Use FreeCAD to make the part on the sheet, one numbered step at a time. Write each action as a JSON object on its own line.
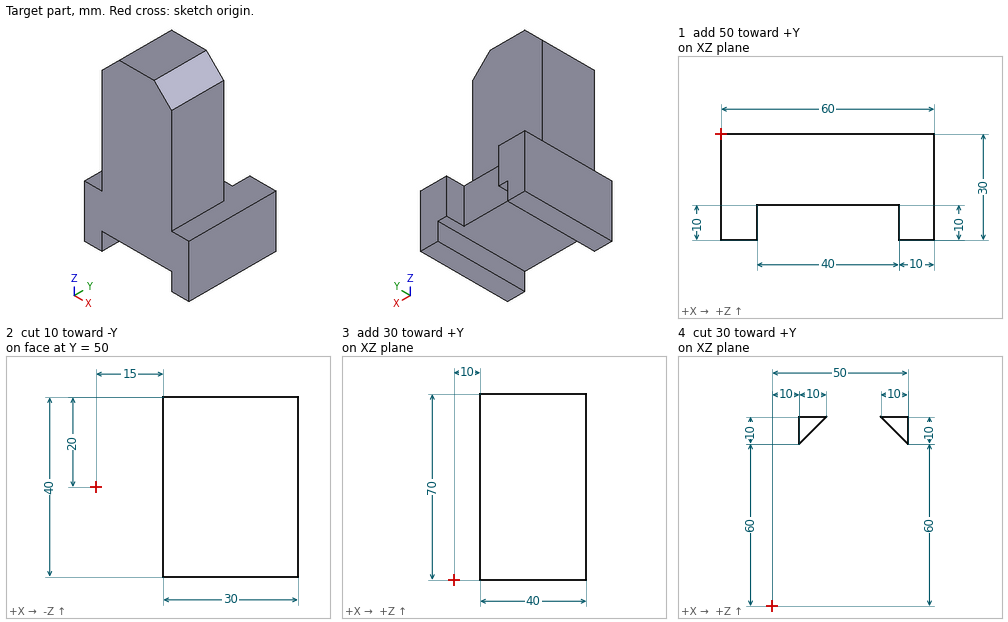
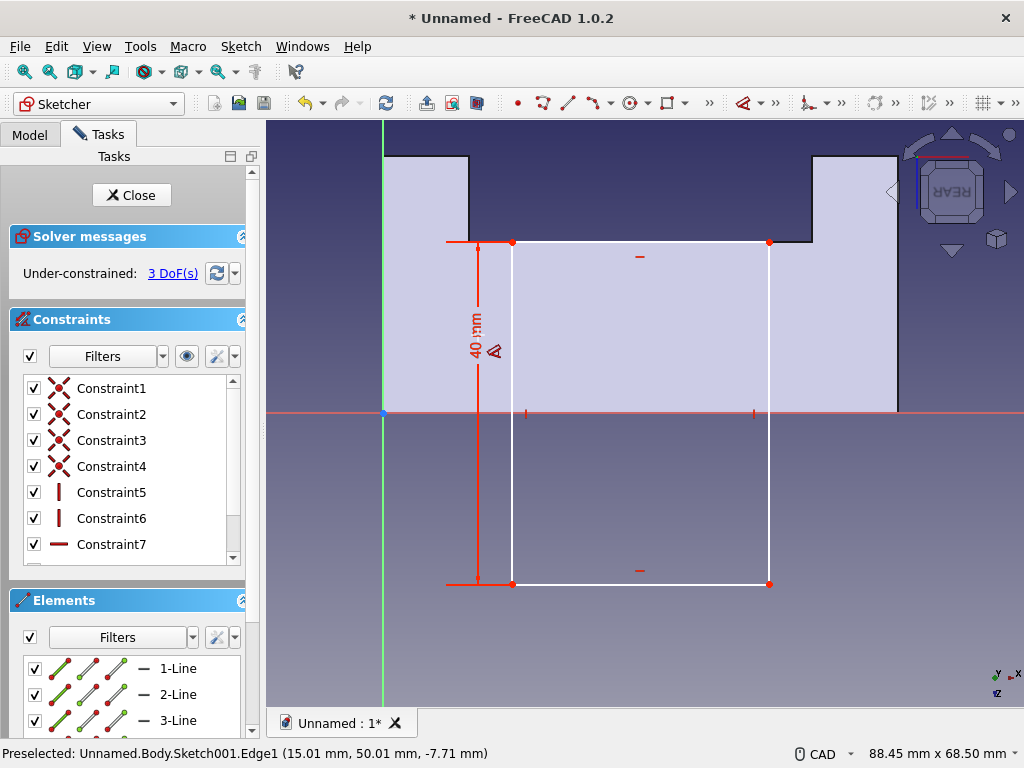
{"action": "left_click", "coordinate": [589, 585]}
{"action": "left_click", "coordinate": [641, 619]}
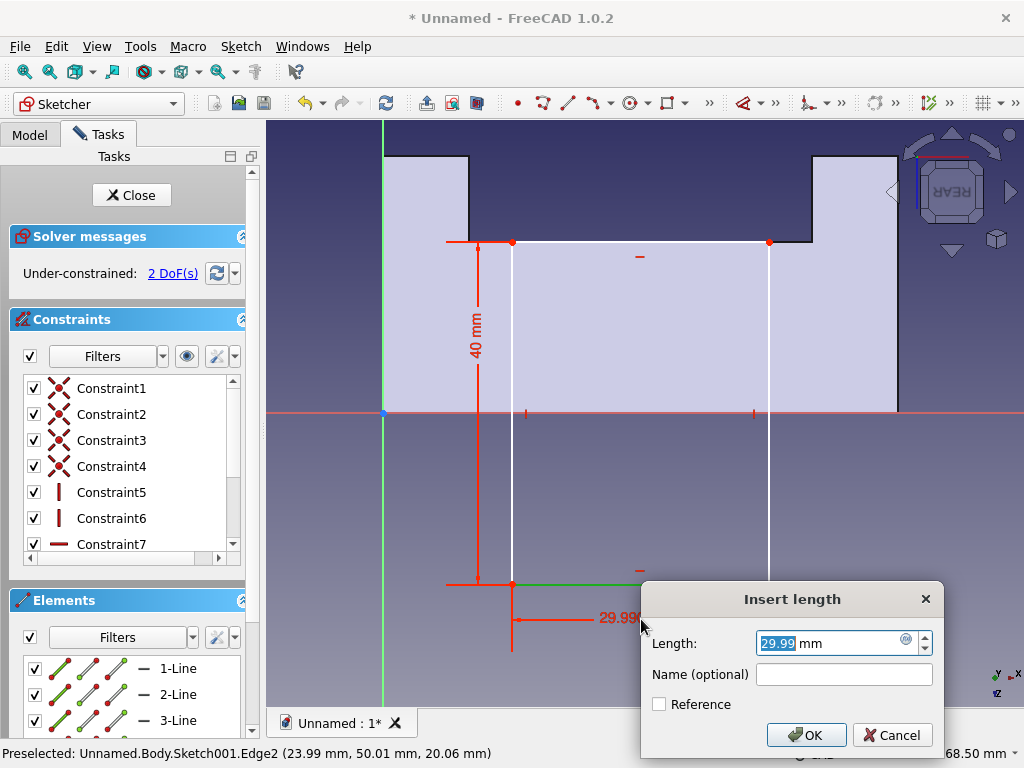
{"action": "type", "text": "30"}
{"action": "key", "text": "Return"}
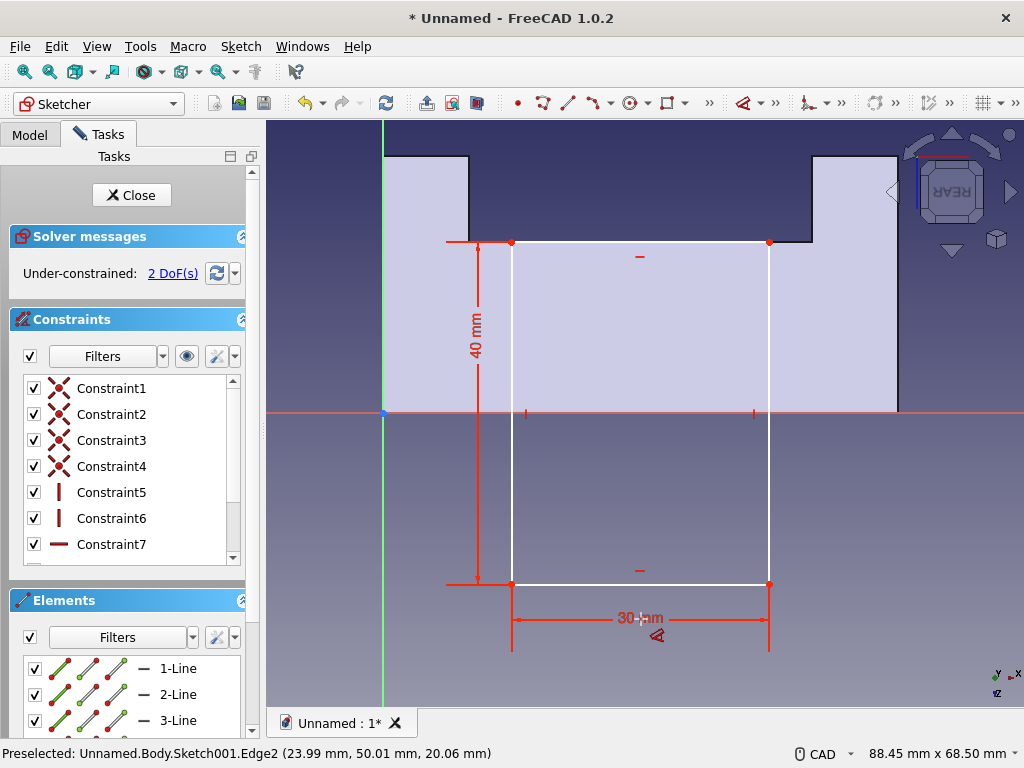
{"action": "left_click", "coordinate": [512, 242]}
{"action": "left_click", "coordinate": [448, 208]}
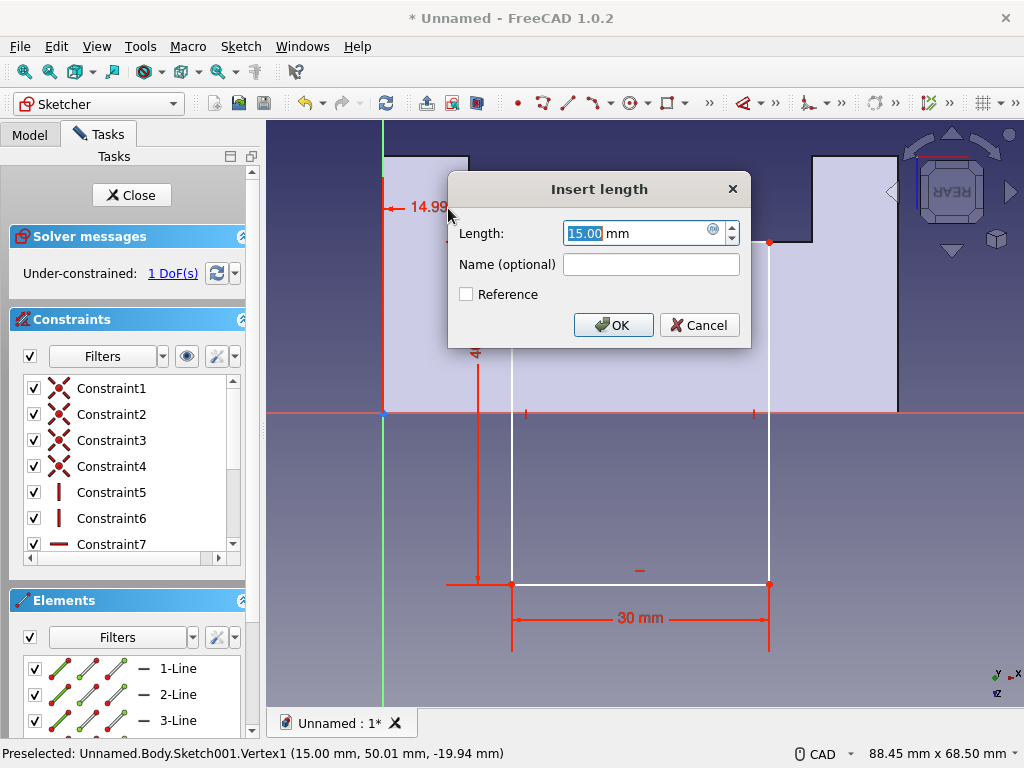
{"action": "type", "text": "15"}
{"action": "key", "text": "Return"}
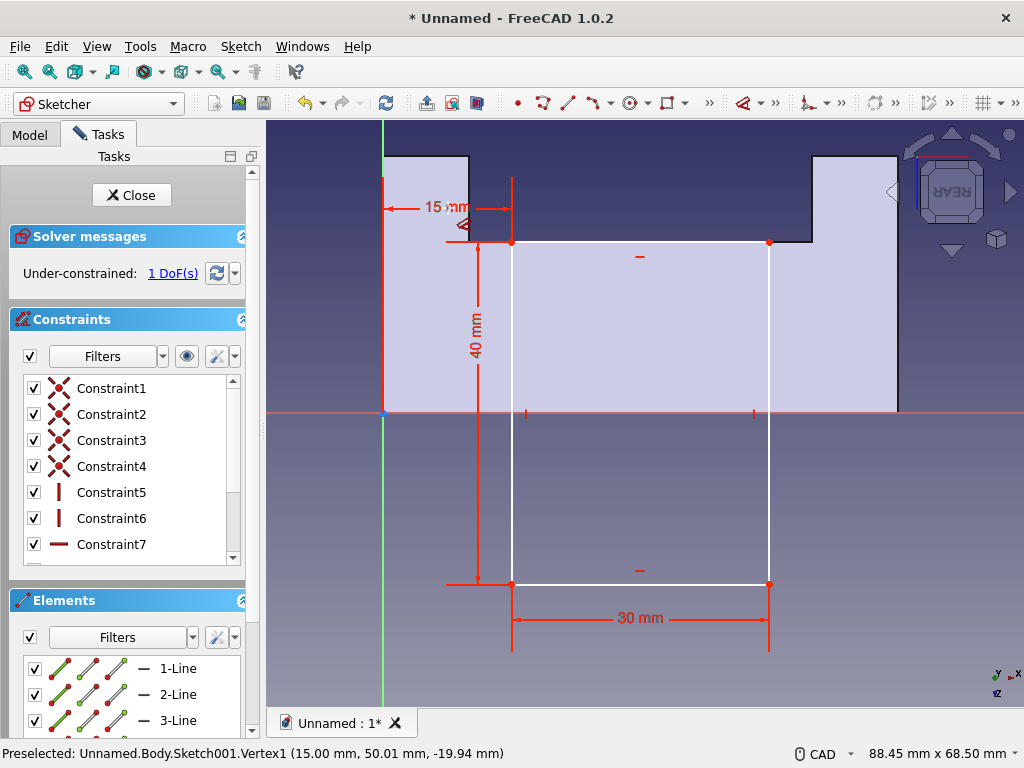
{"action": "left_click", "coordinate": [512, 242]}
{"action": "left_click", "coordinate": [349, 328]}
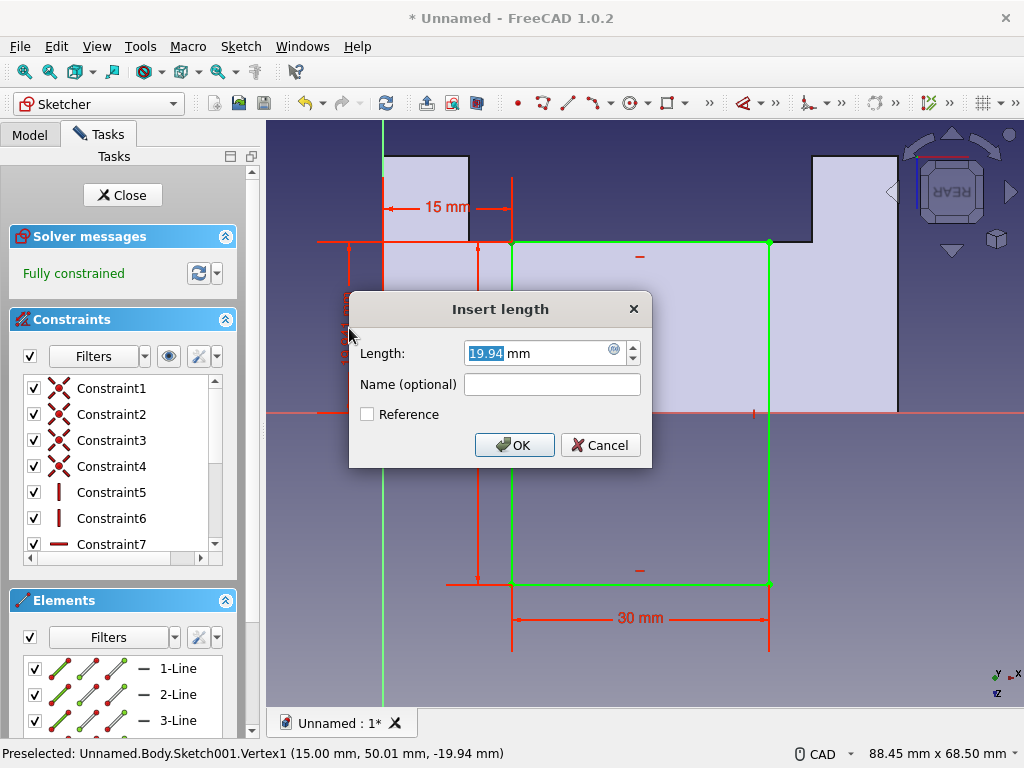
{"action": "type", "text": "20"}
{"action": "key", "text": "Return"}
{"action": "key", "text": "Escape"}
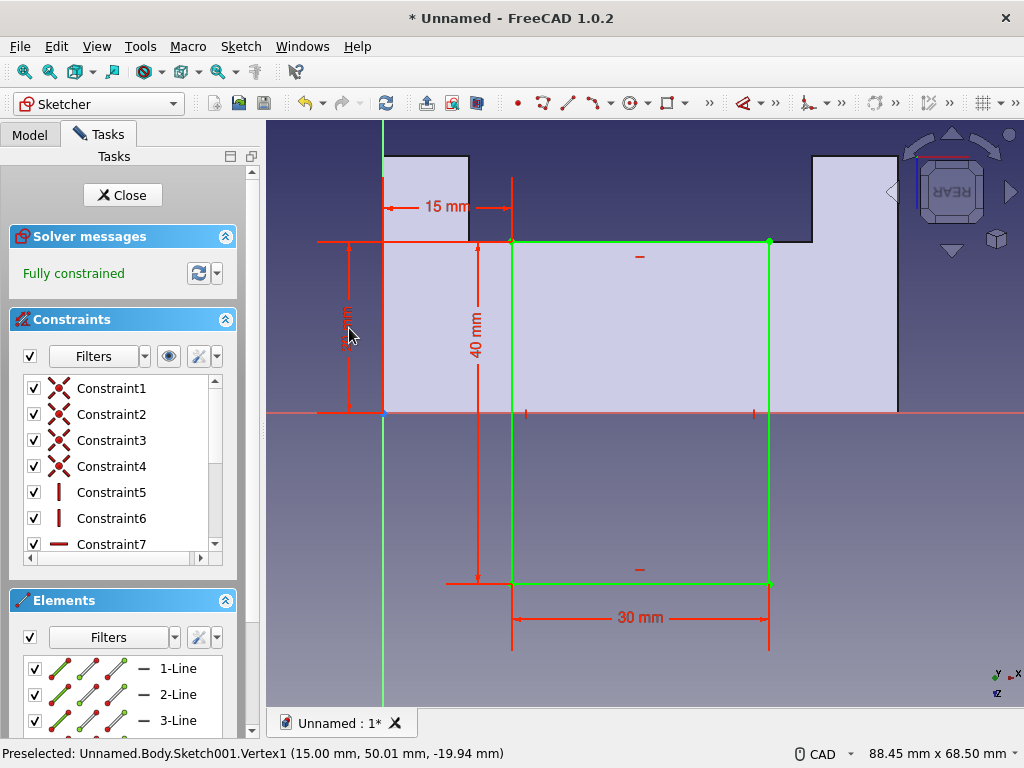
{"action": "left_click", "coordinate": [123, 195]}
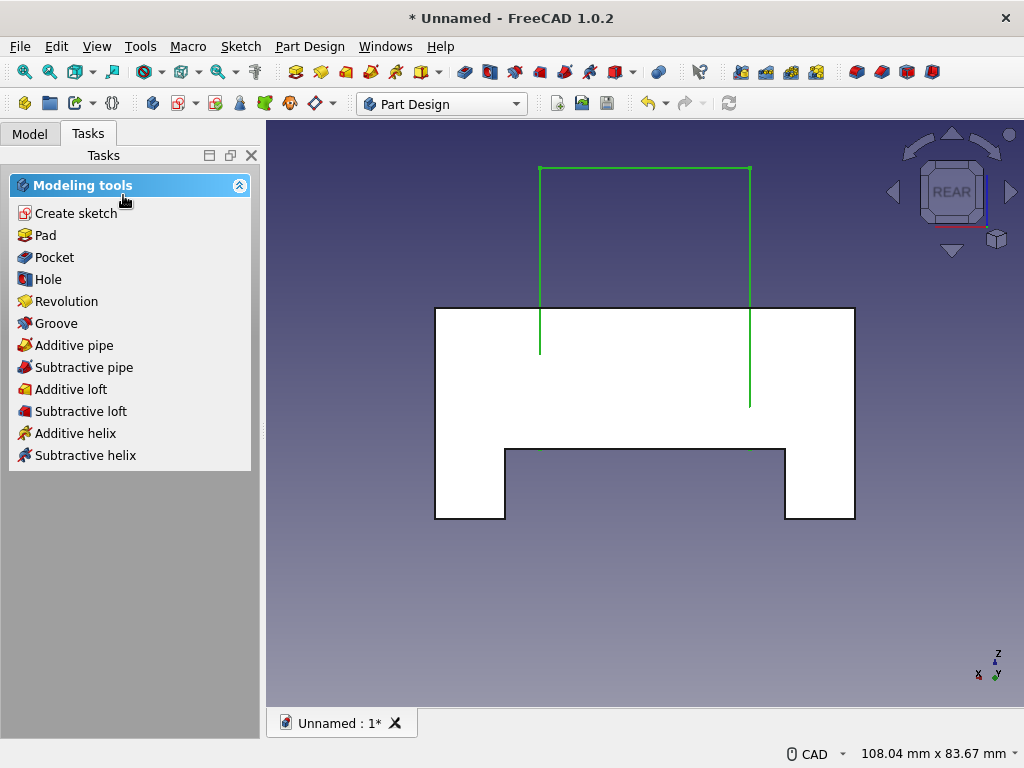
{"action": "left_click", "coordinate": [465, 72]}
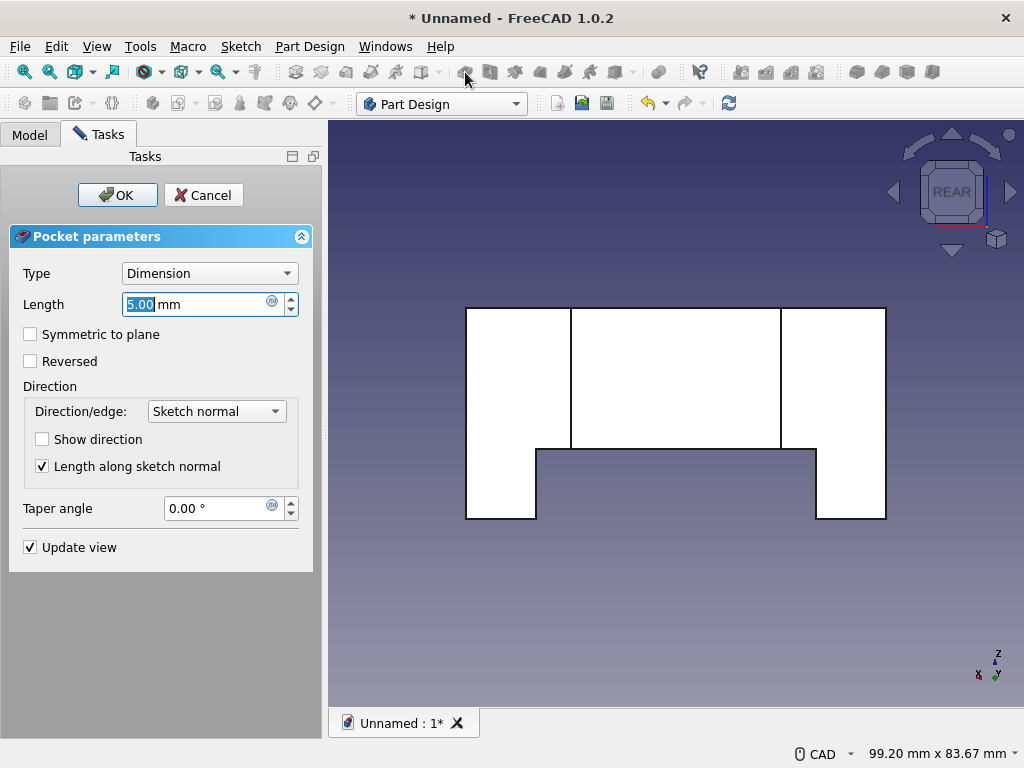
{"action": "type", "text": "10"}
{"action": "key", "text": "Tab"}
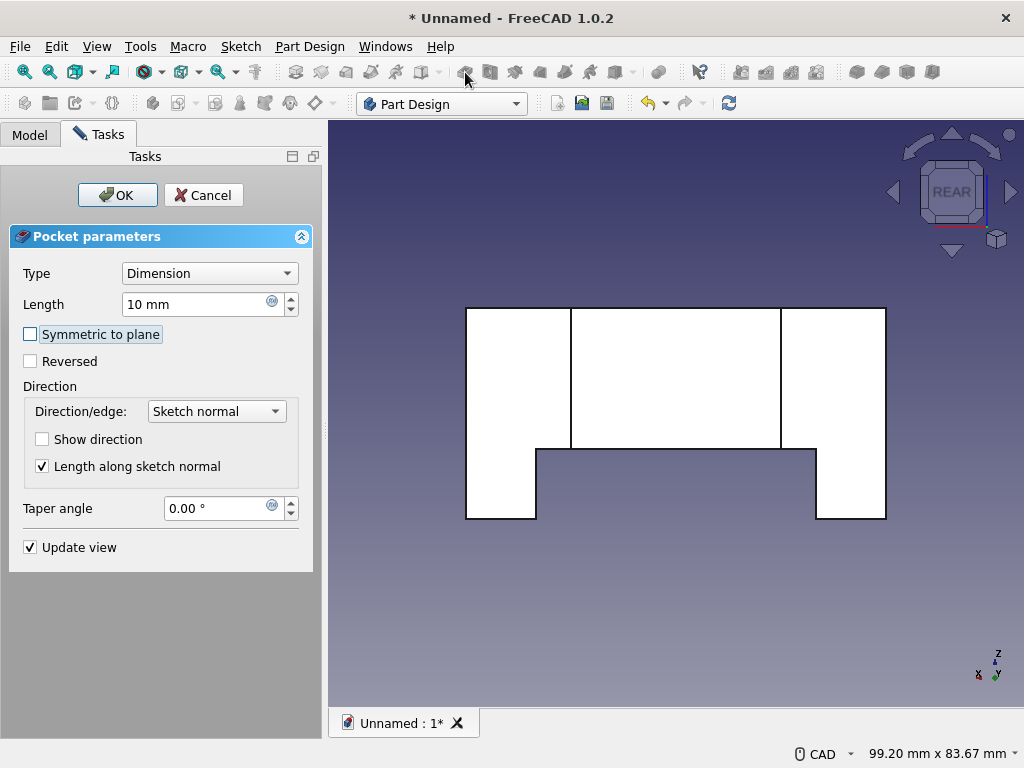
{"action": "left_click", "coordinate": [118, 195]}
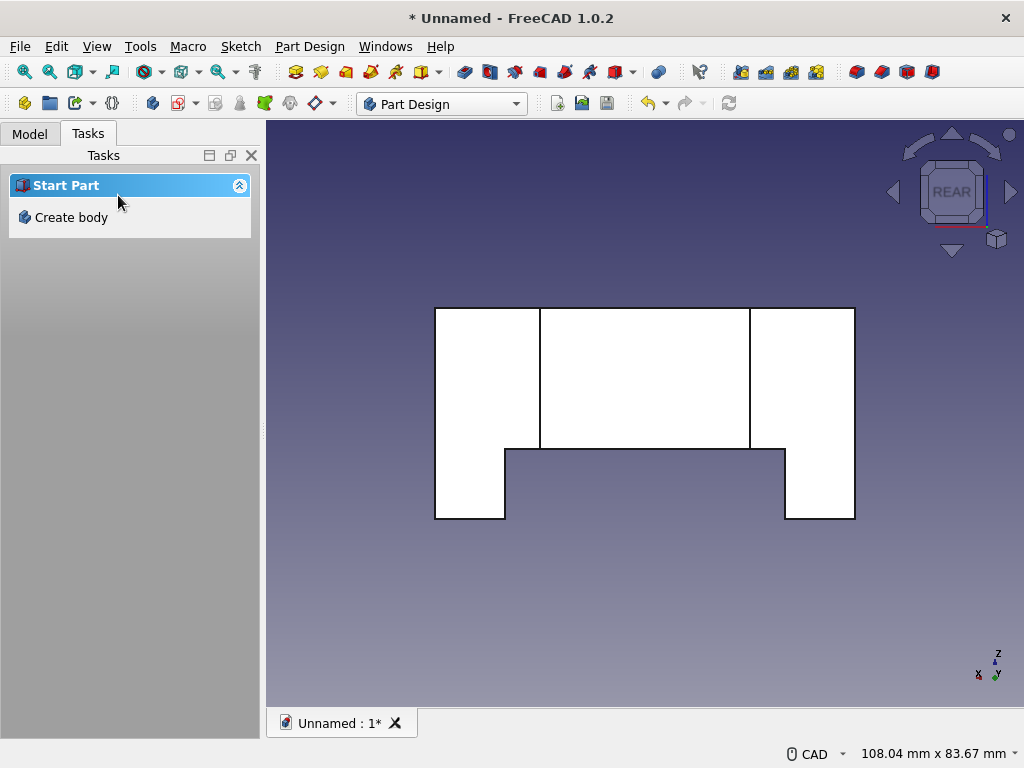
{"action": "left_click", "coordinate": [178, 104]}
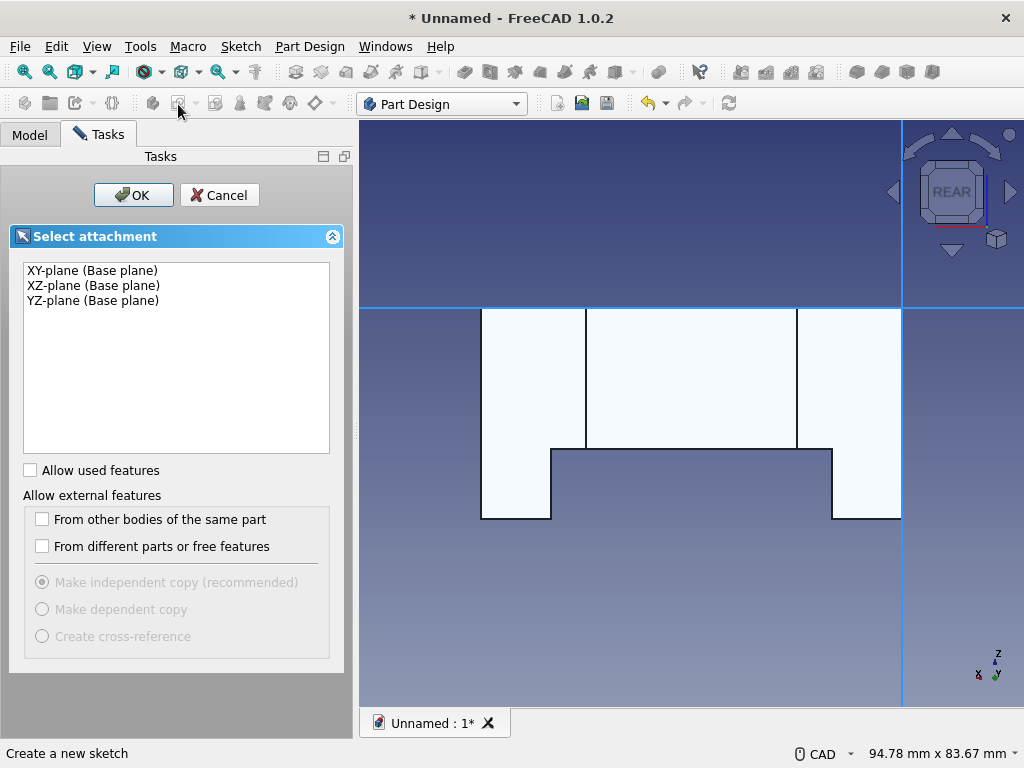
{"action": "left_click", "coordinate": [84, 286]}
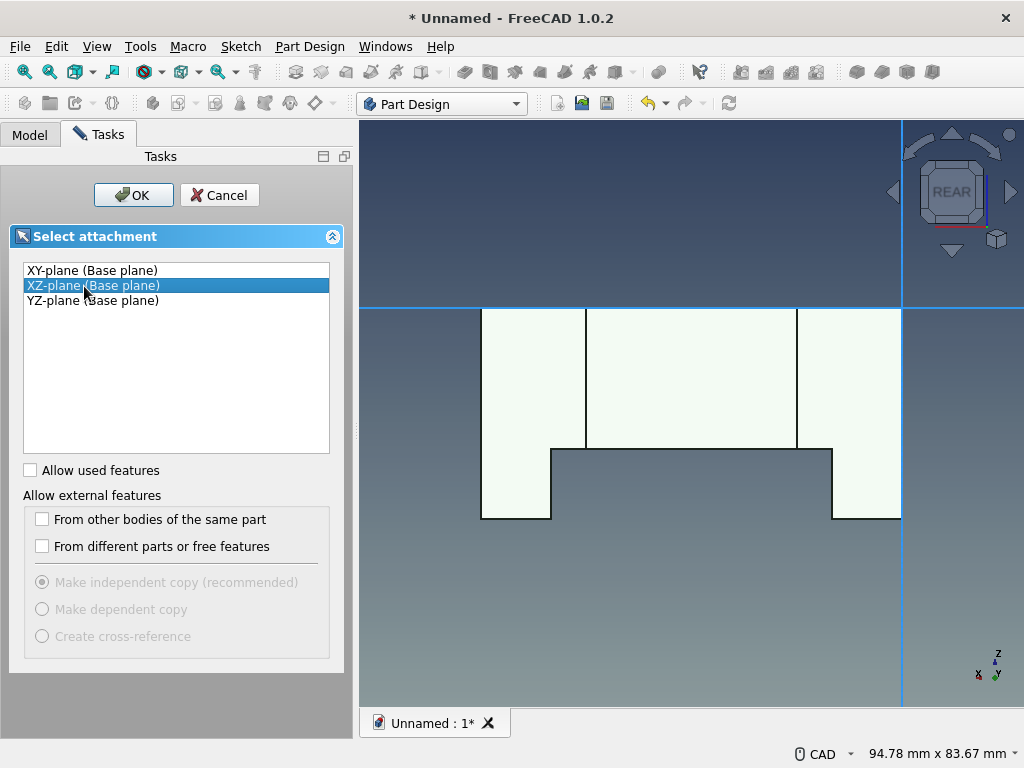
{"action": "left_click", "coordinate": [134, 195]}